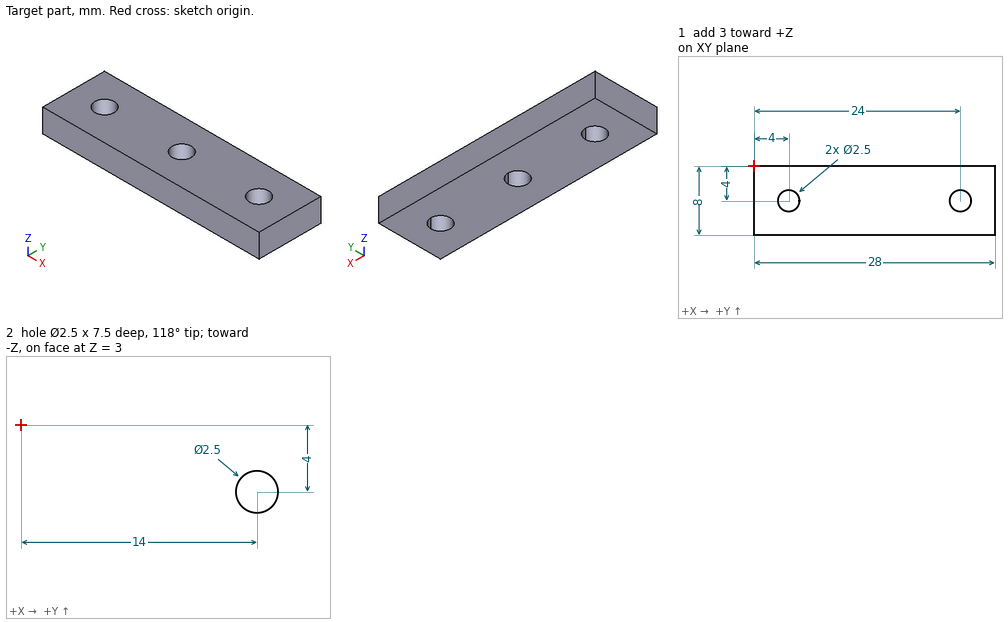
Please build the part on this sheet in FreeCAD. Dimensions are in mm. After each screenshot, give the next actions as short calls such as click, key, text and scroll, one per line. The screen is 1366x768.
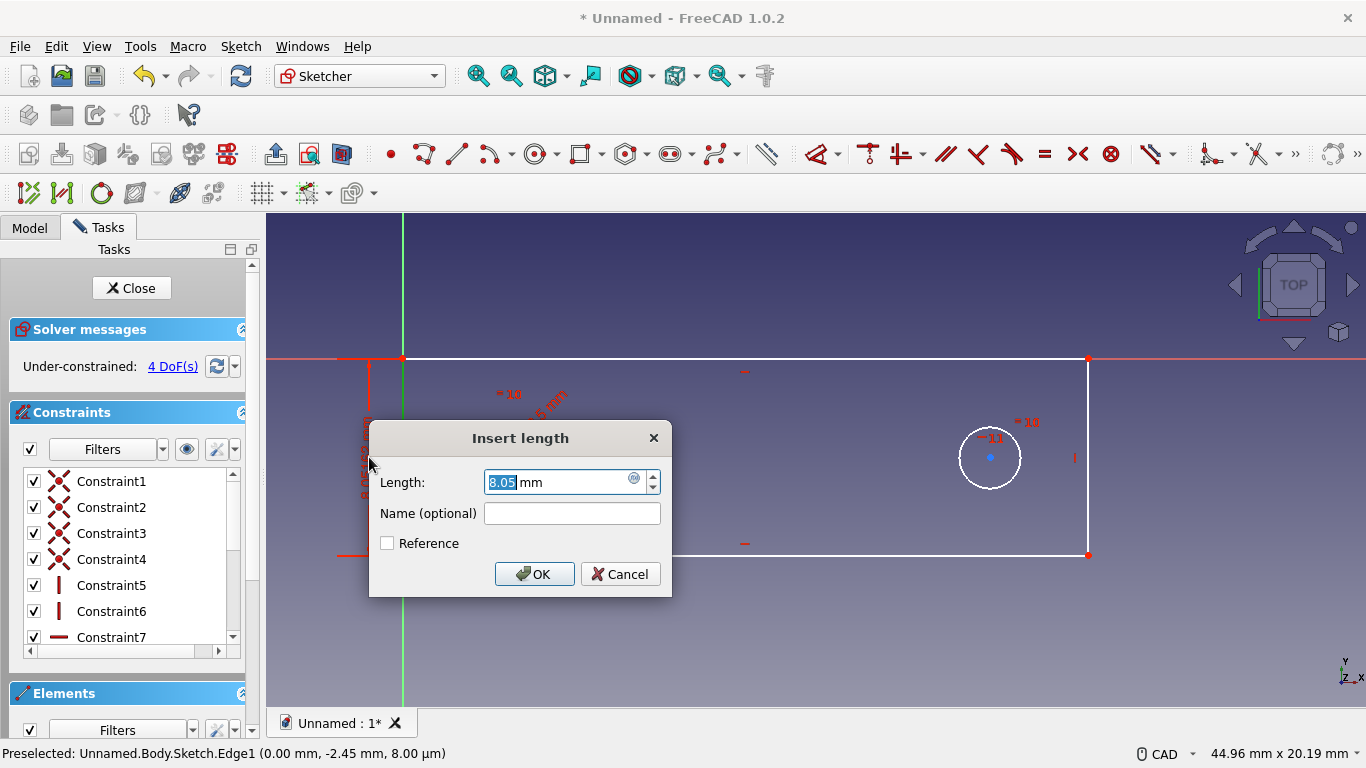
text(8)
key(Return)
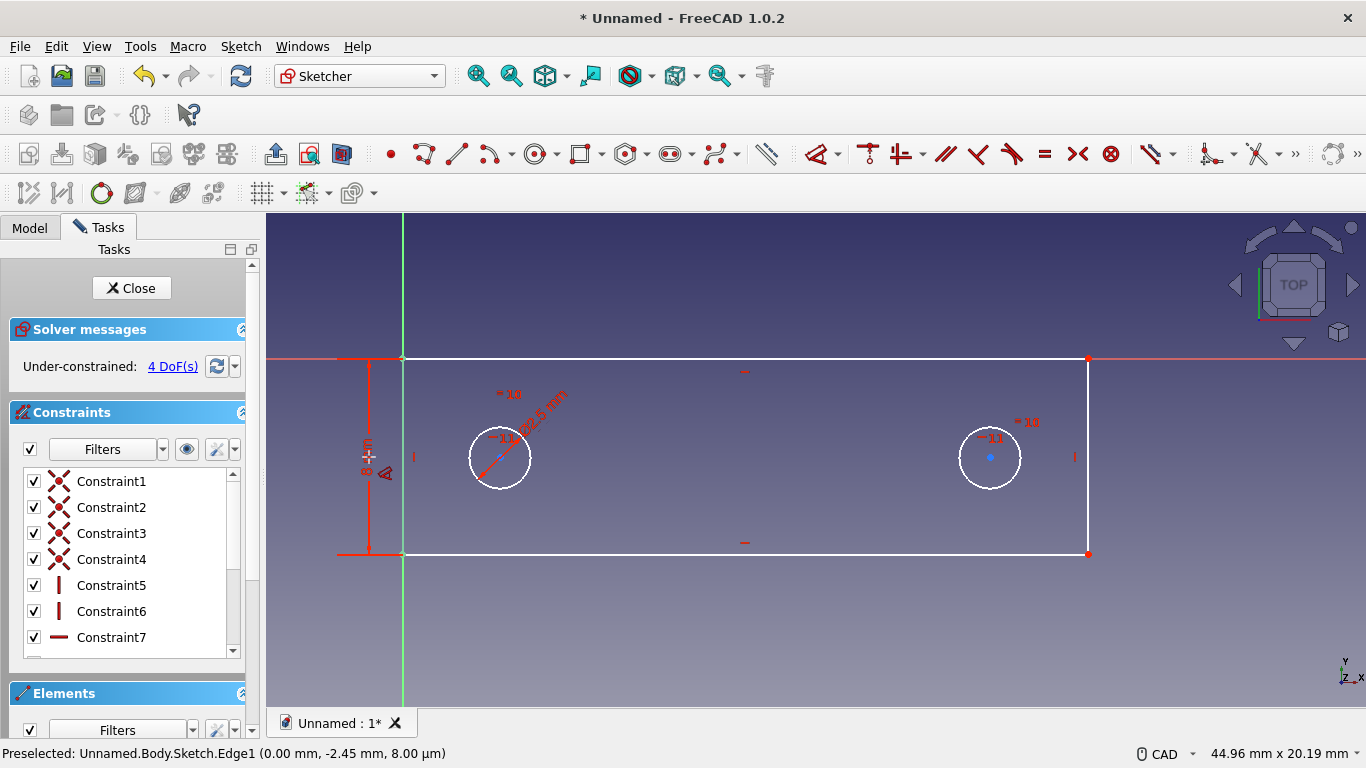
click(500, 458)
click(451, 325)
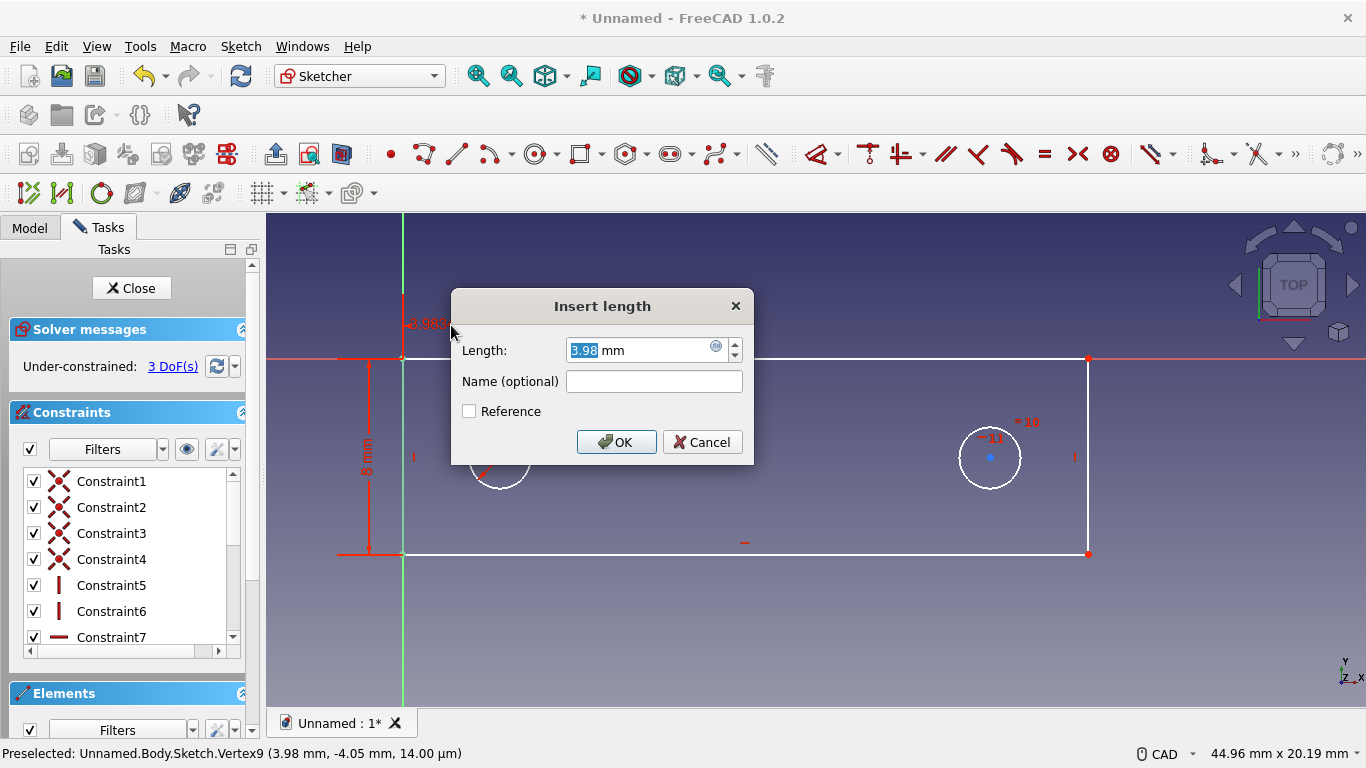
text(4)
key(Return)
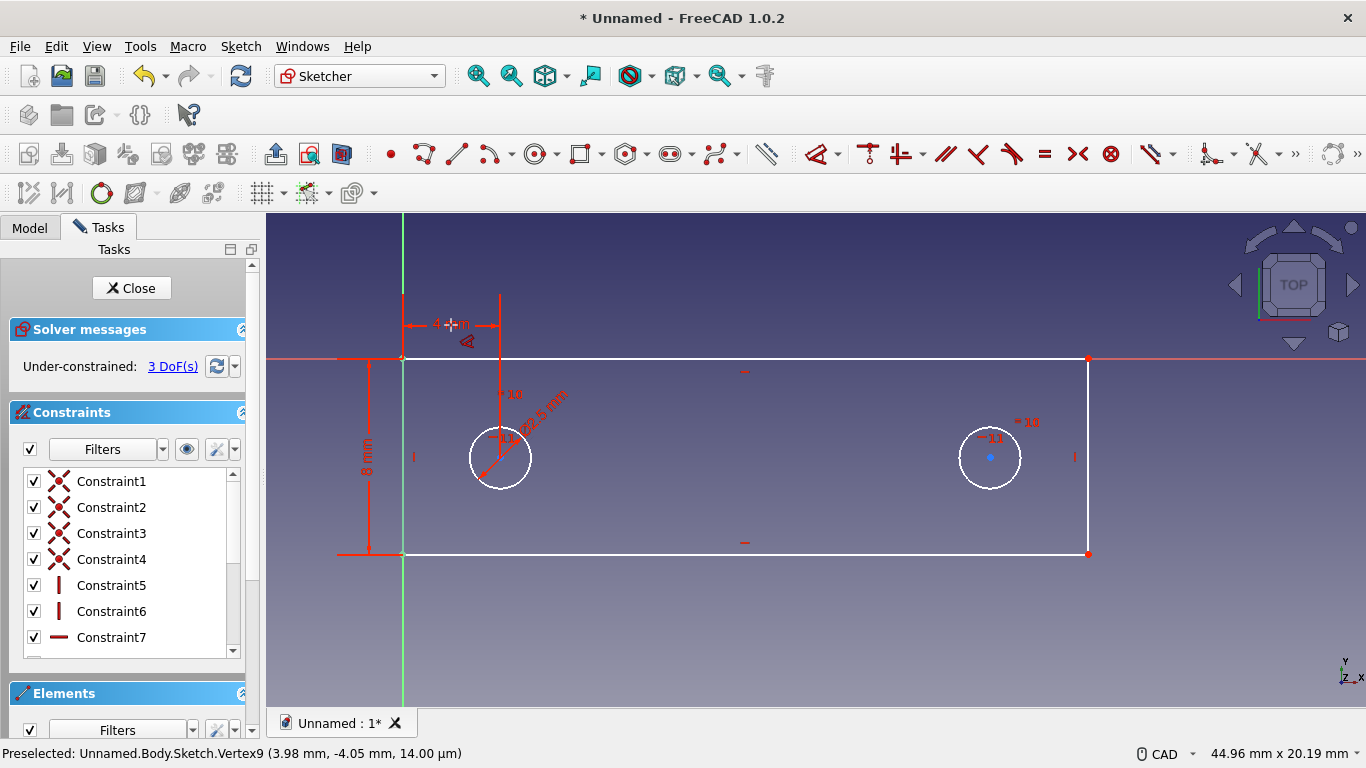
click(500, 458)
click(369, 408)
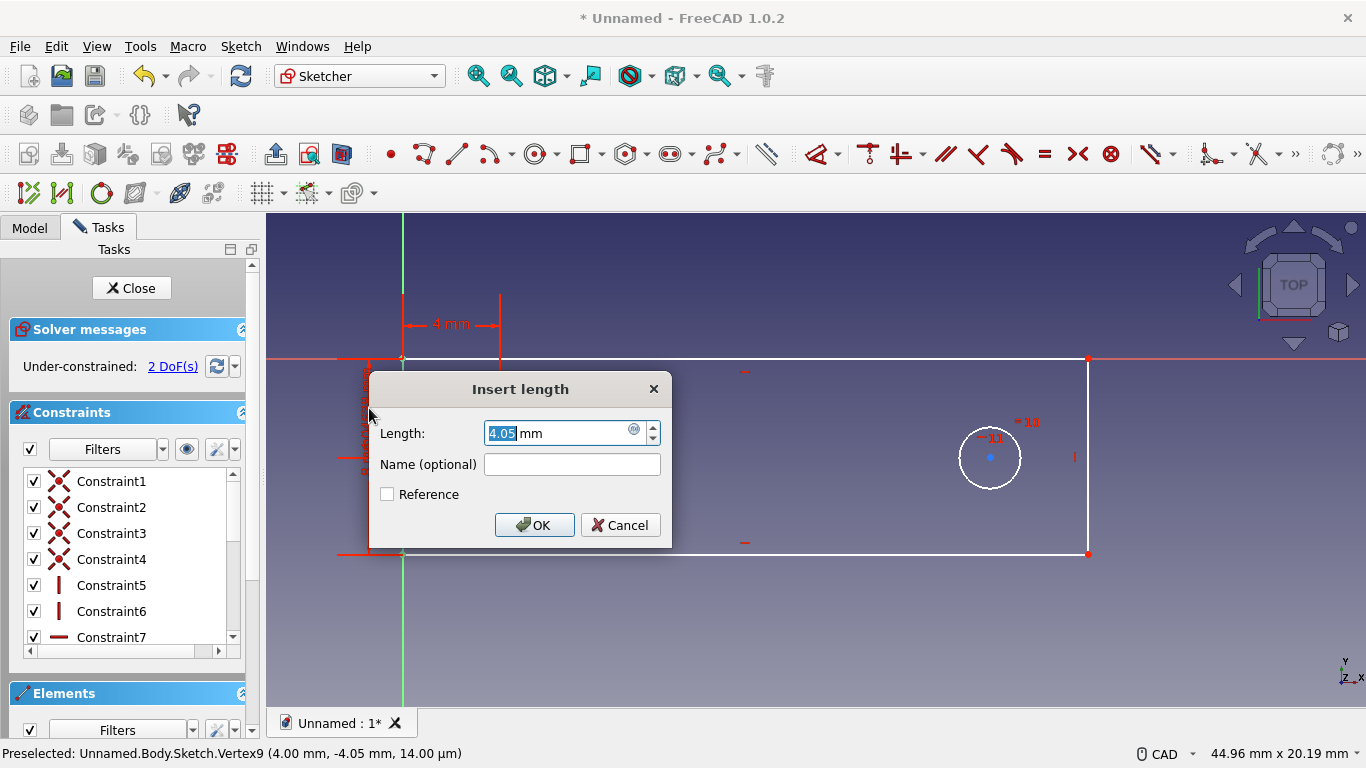
text(4)
key(Return)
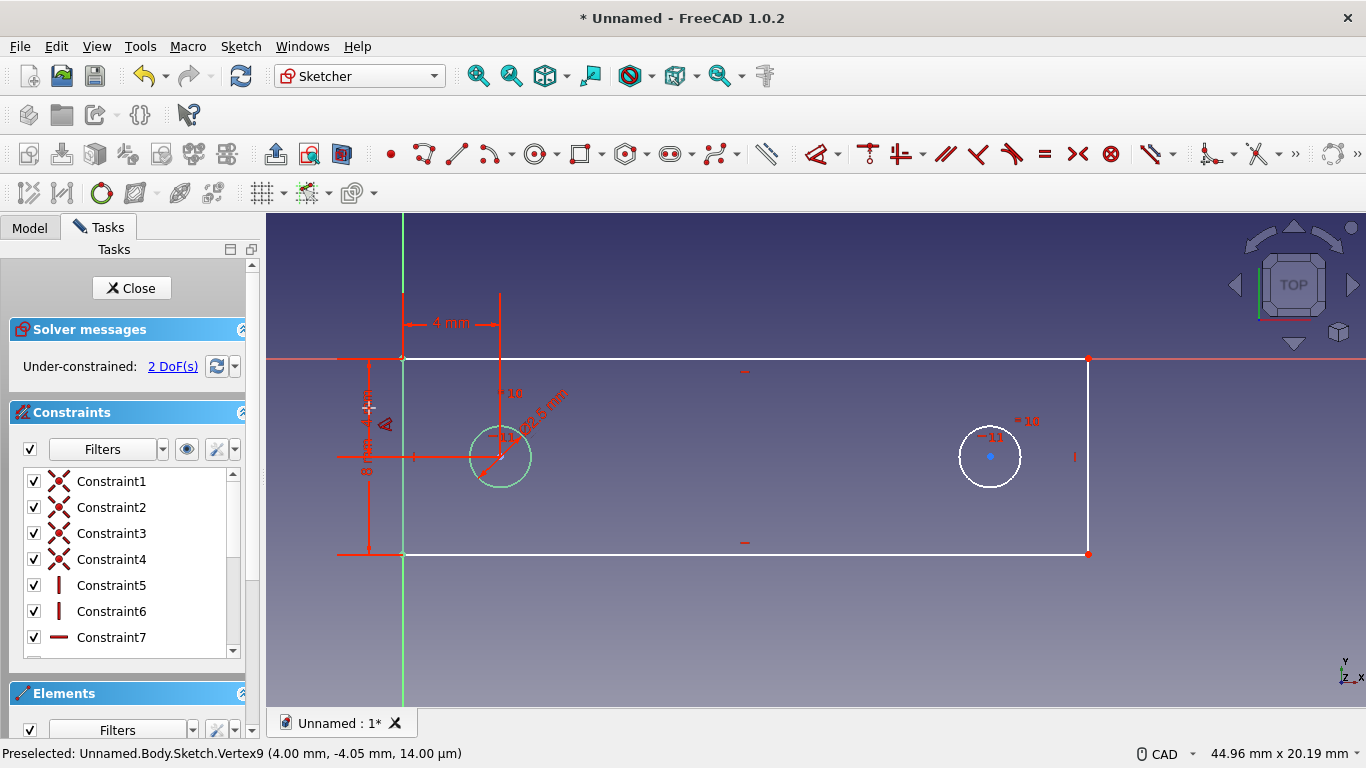
click(608, 555)
click(745, 589)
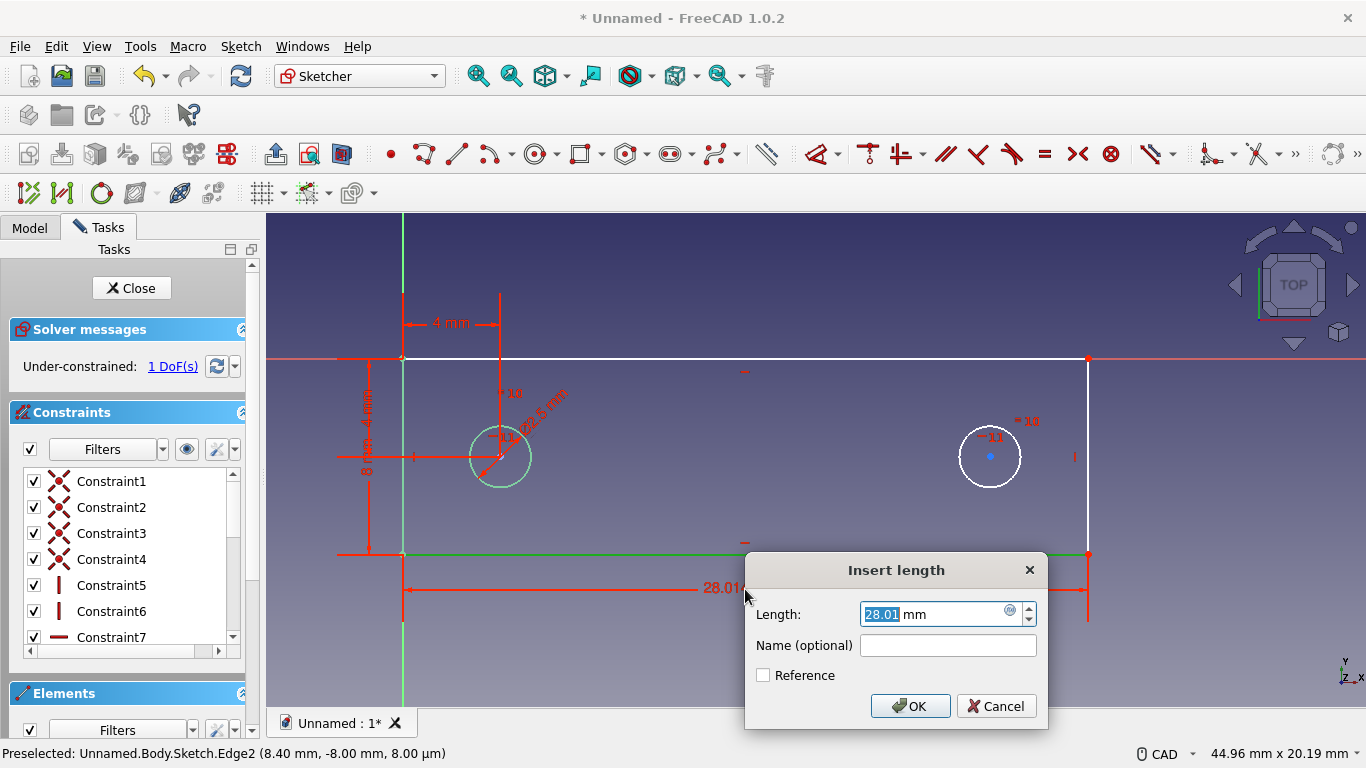
text(28)
key(Return)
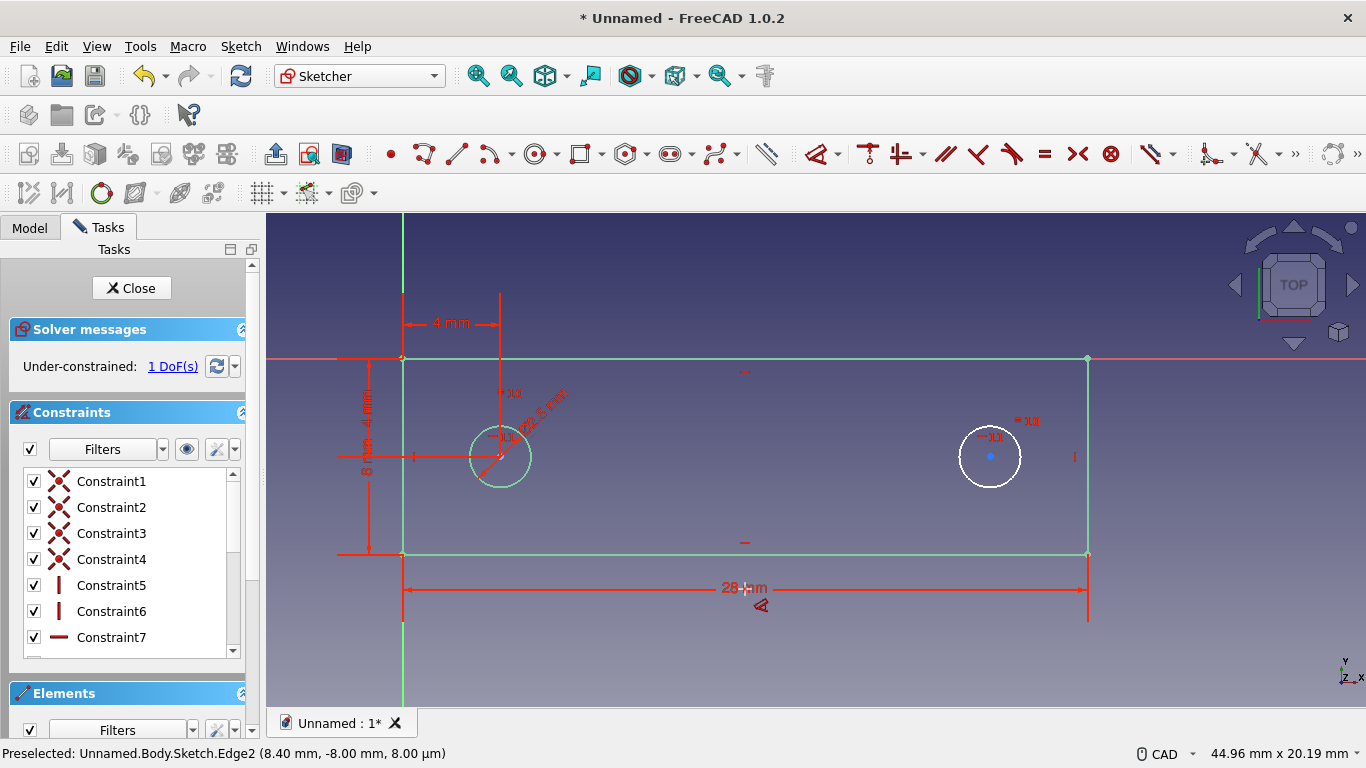
click(990, 457)
click(696, 325)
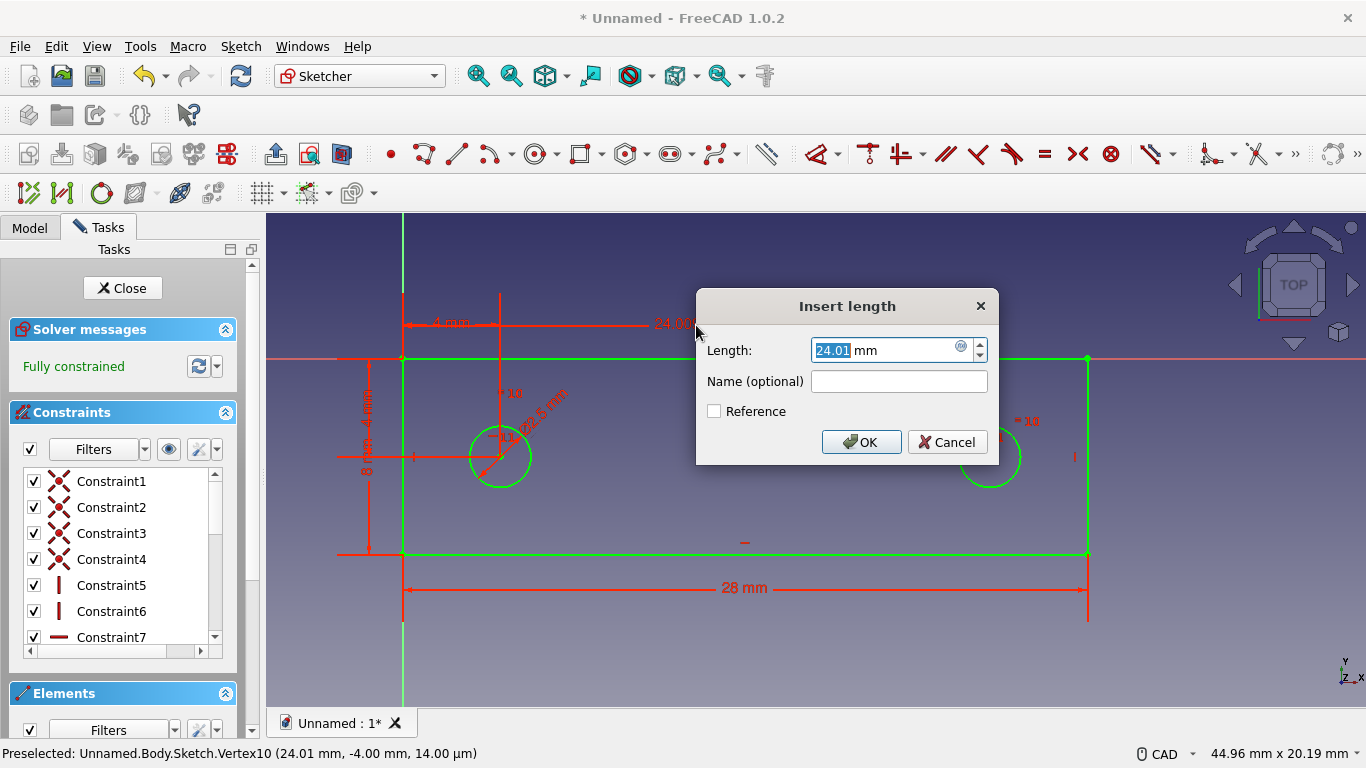
text(24)
key(Return)
key(Escape)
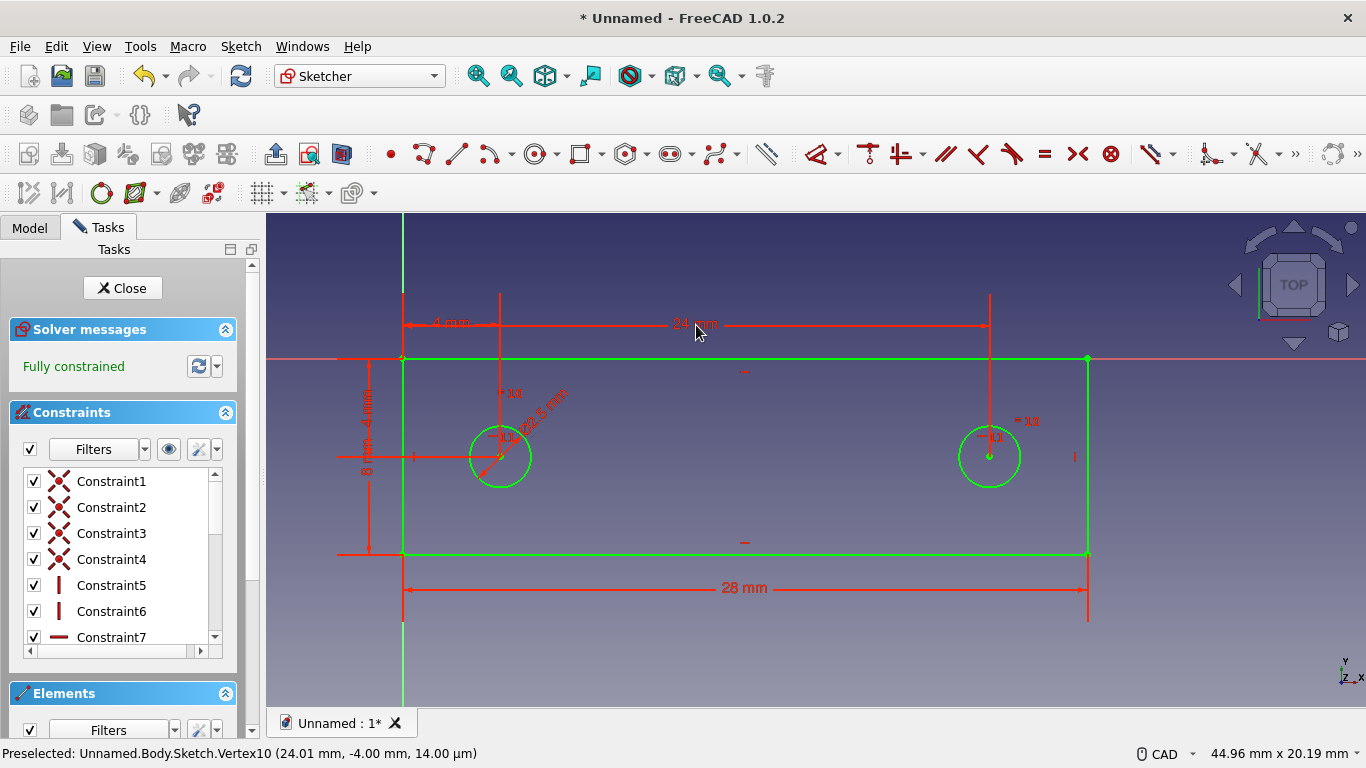
click(123, 288)